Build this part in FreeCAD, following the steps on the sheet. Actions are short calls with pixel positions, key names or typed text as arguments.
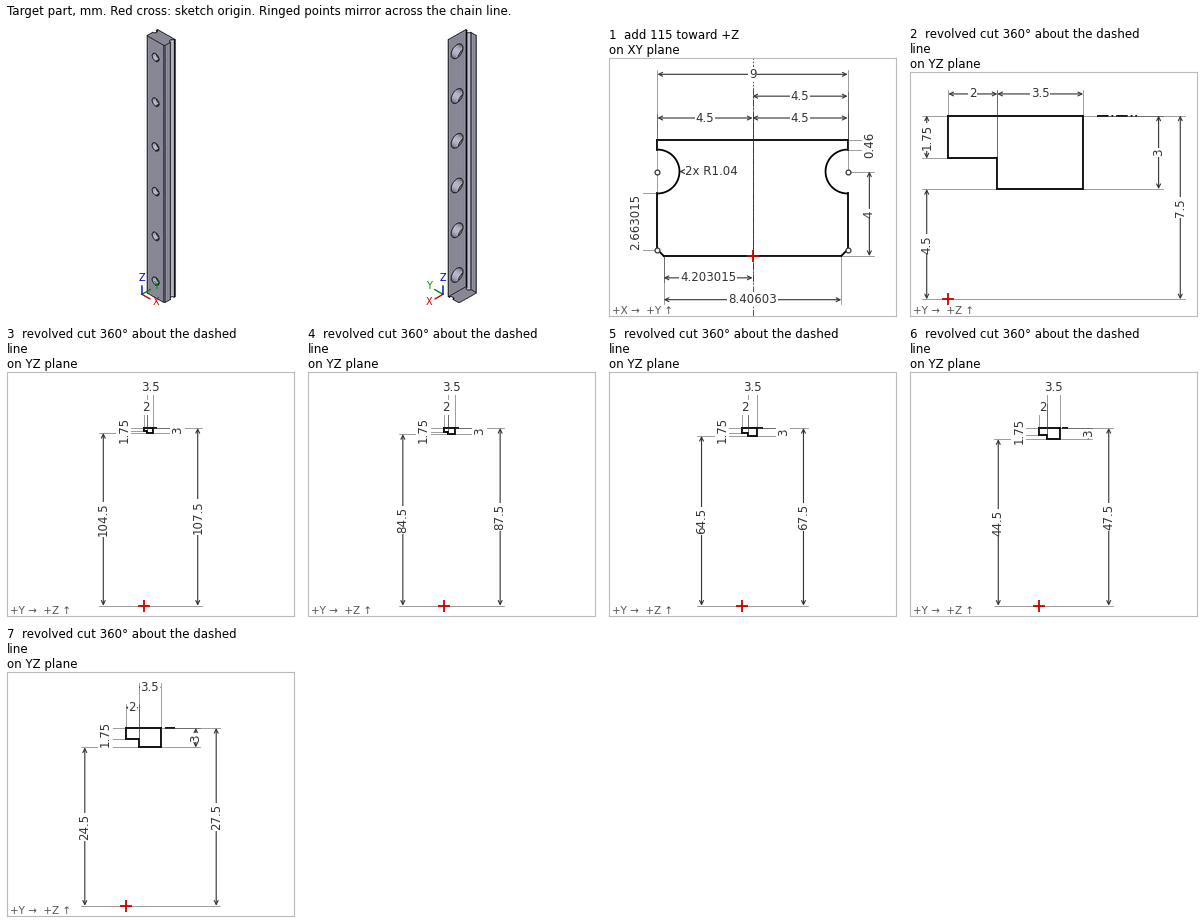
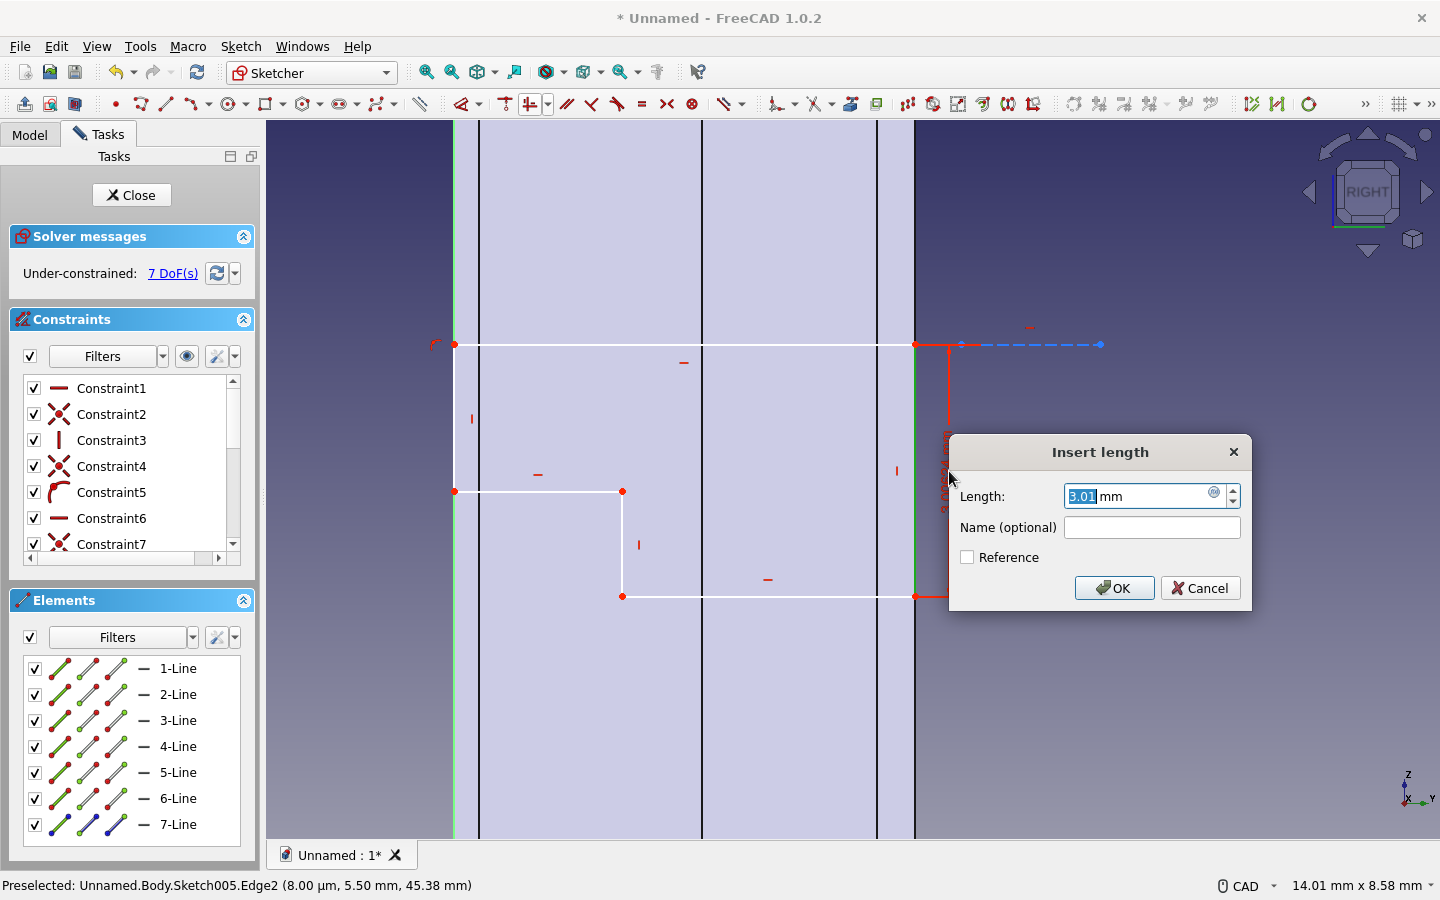
text(3)
key(Return)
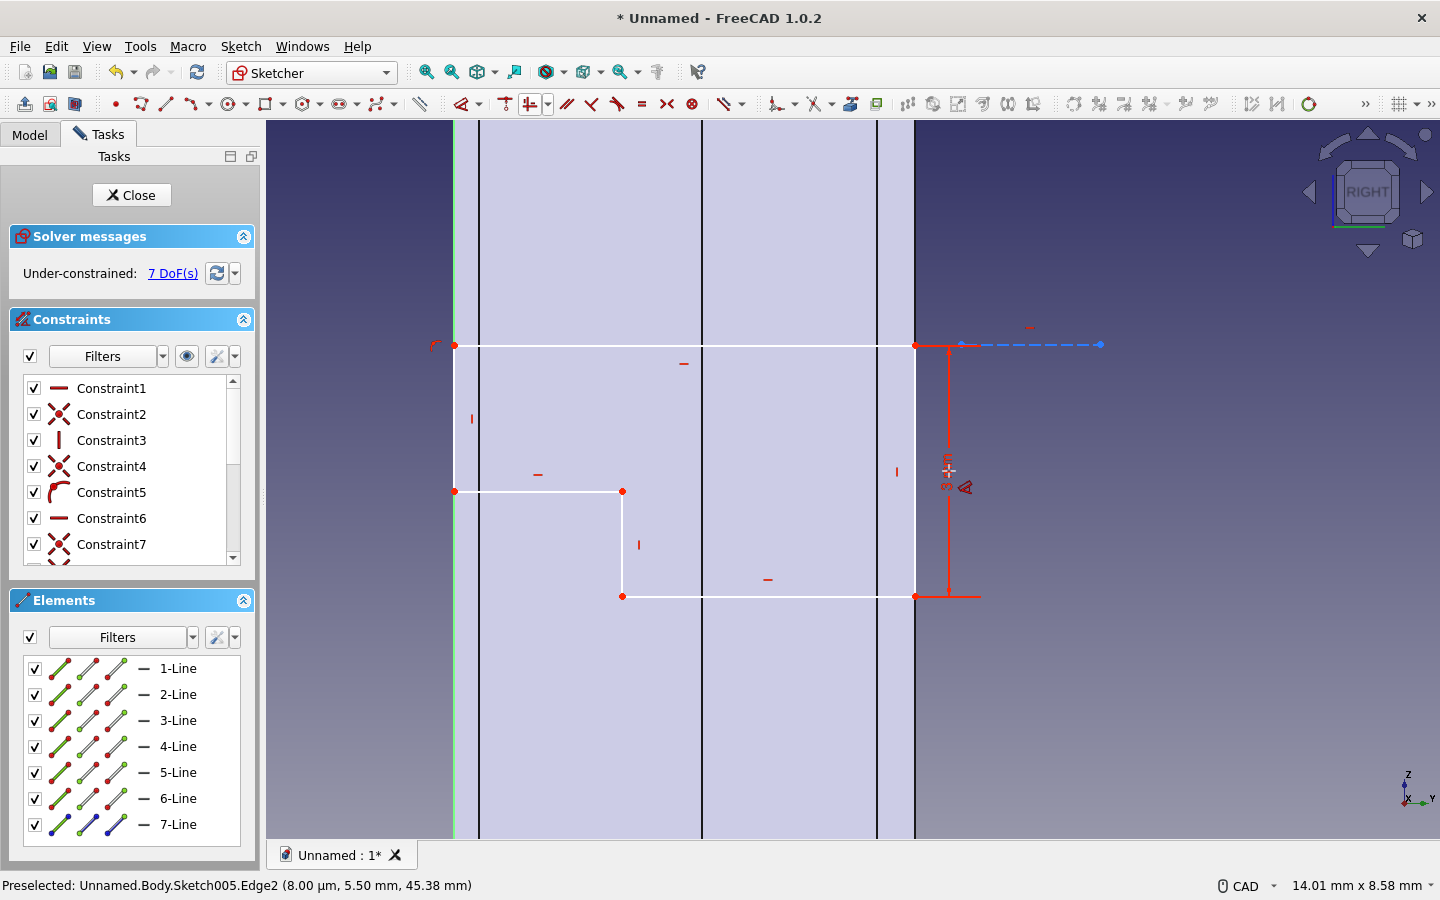
click(504, 492)
click(538, 526)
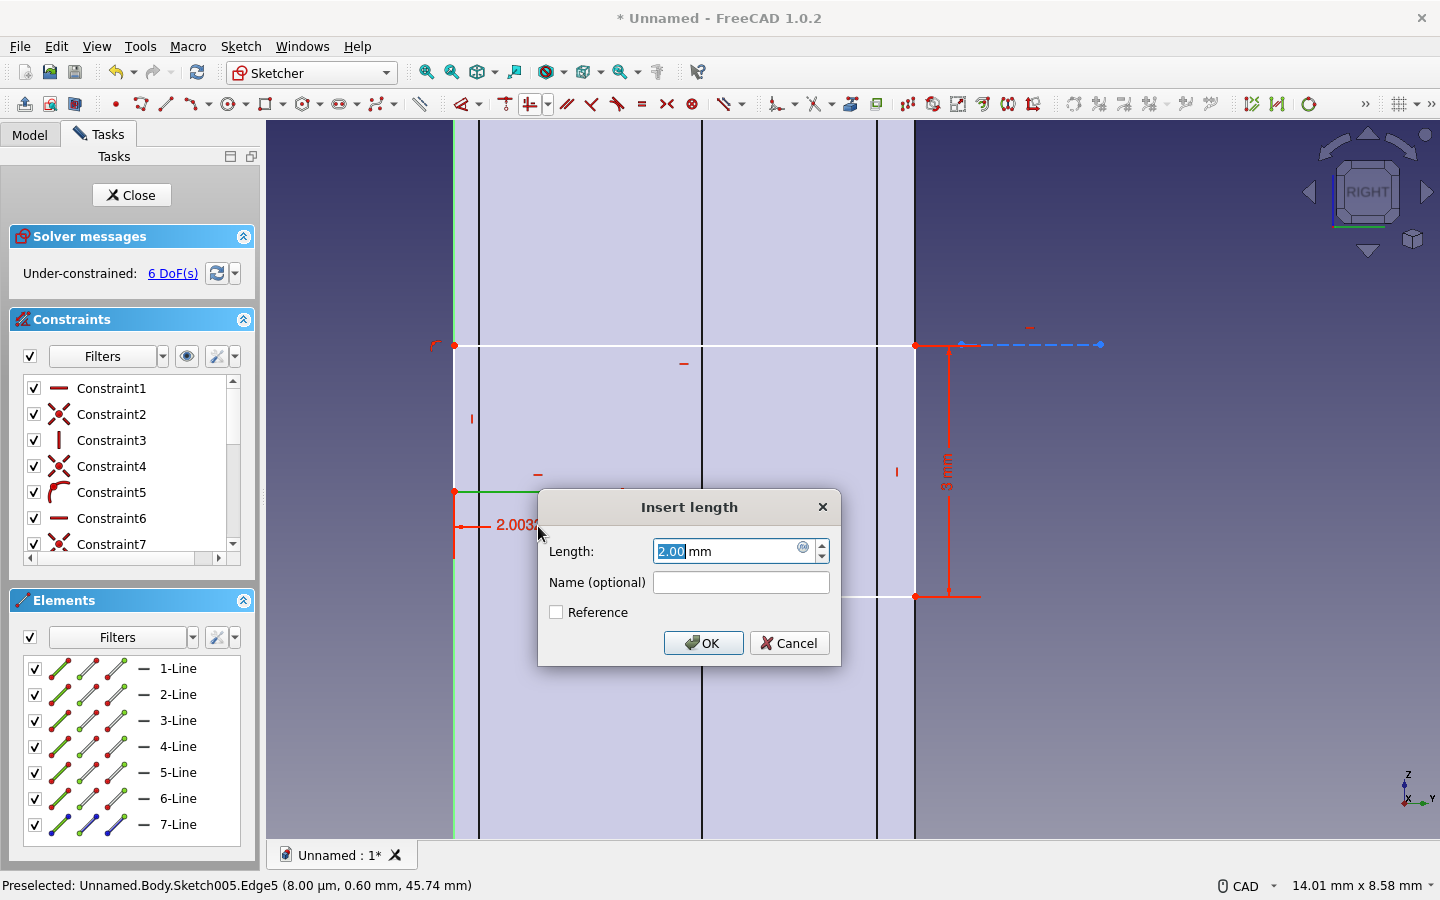
text(2)
key(Return)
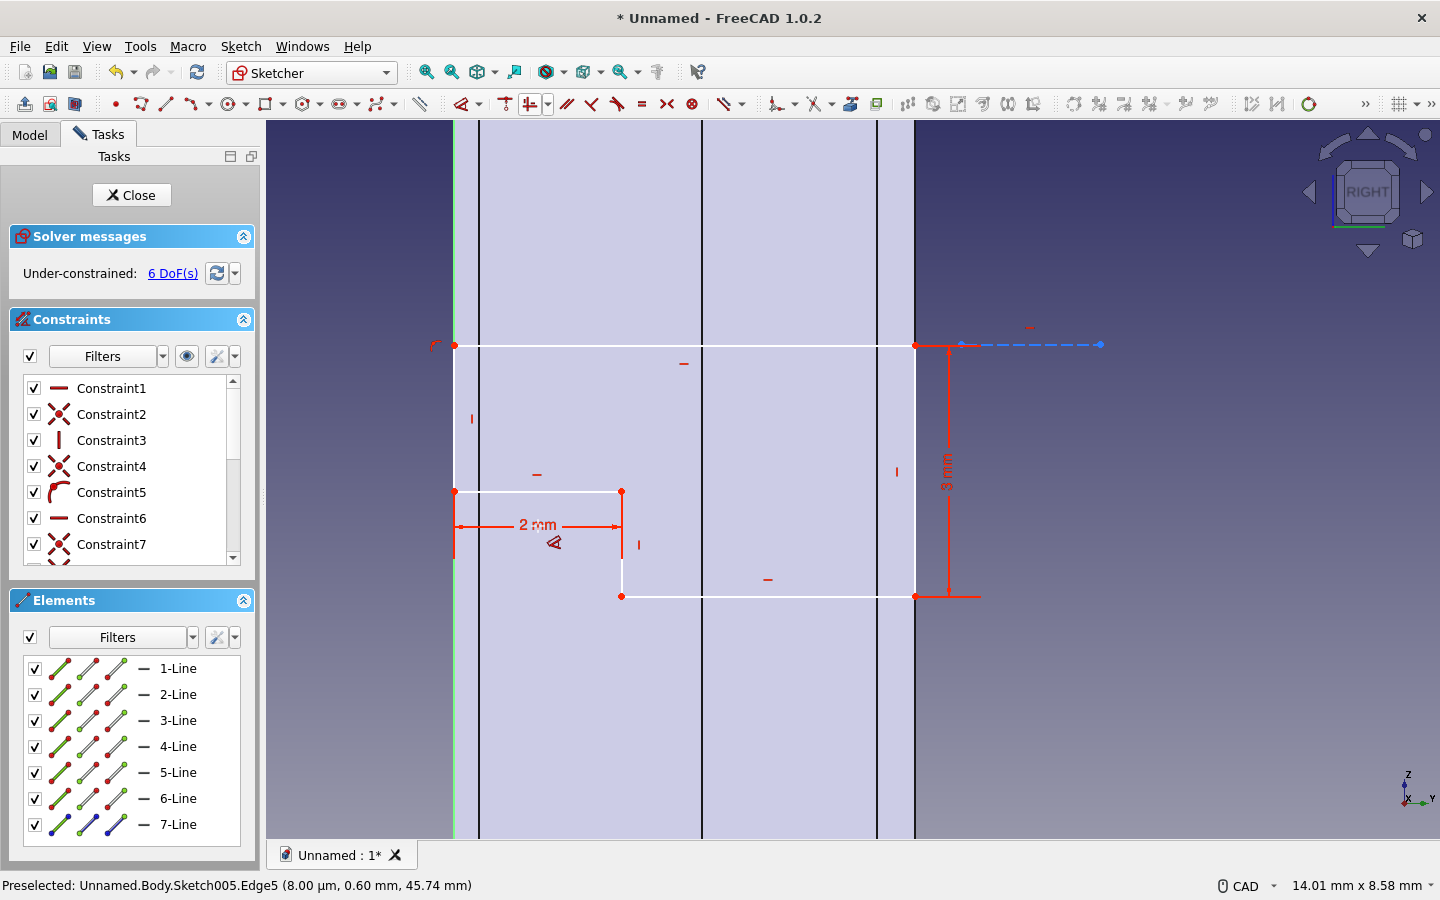
click(710, 597)
click(768, 631)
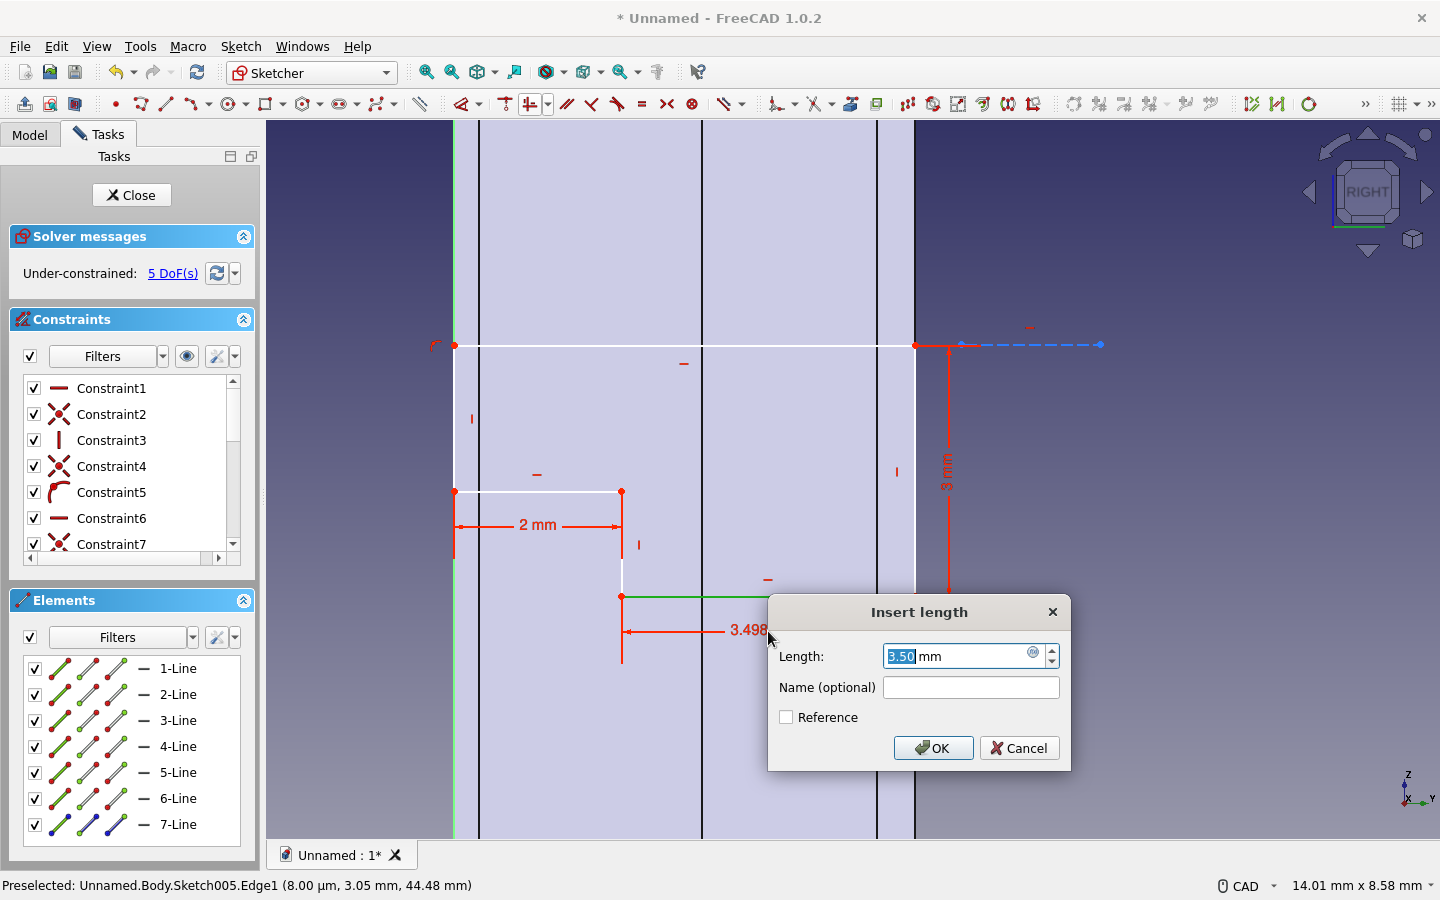
text(3.5)
key(Return)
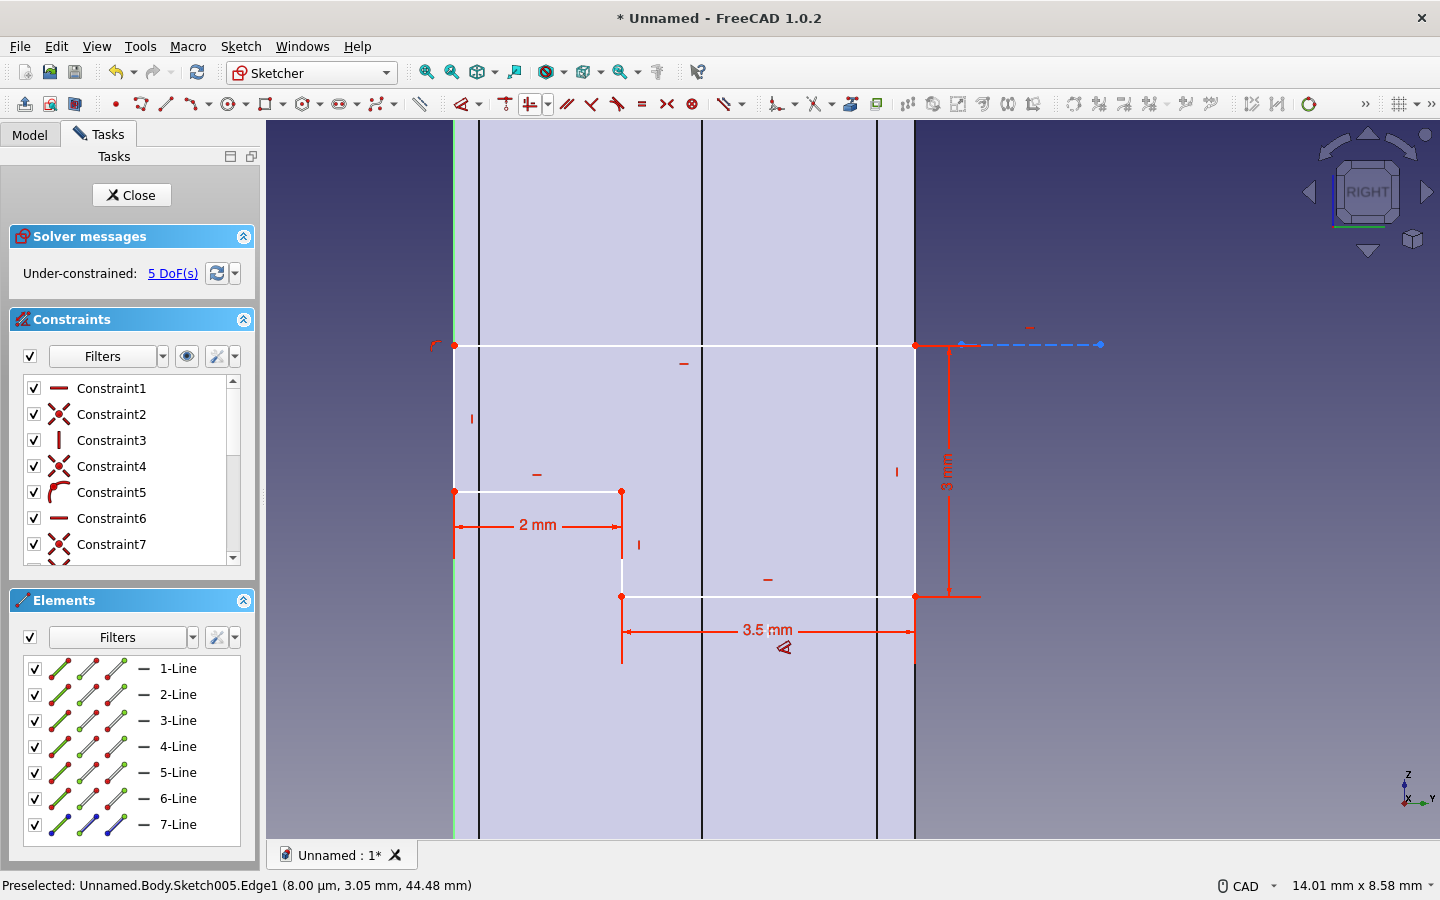
click(454, 389)
click(420, 419)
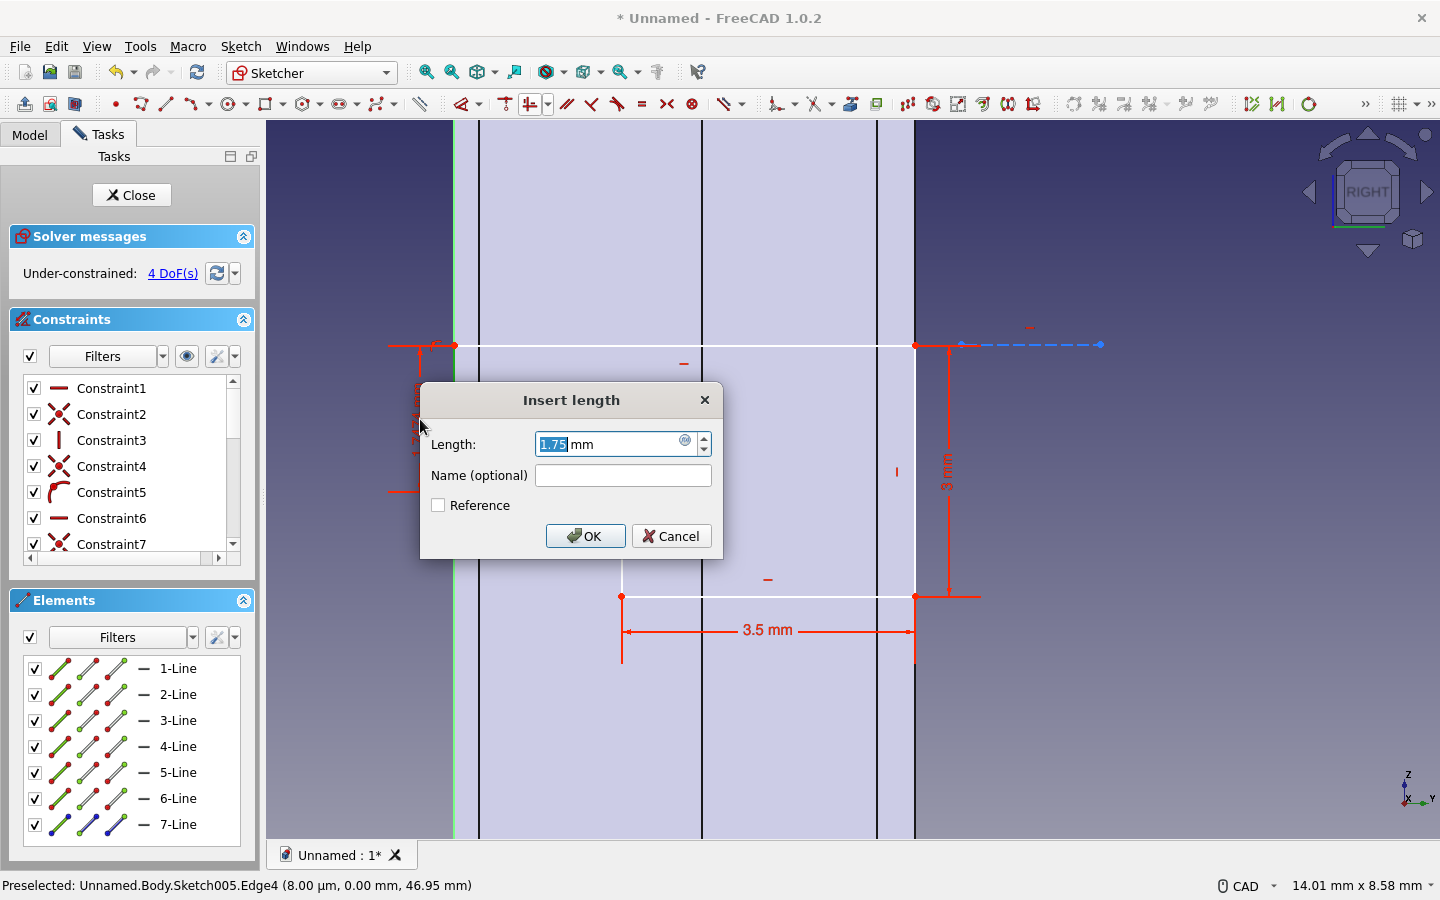
text(1.75)
key(Return)